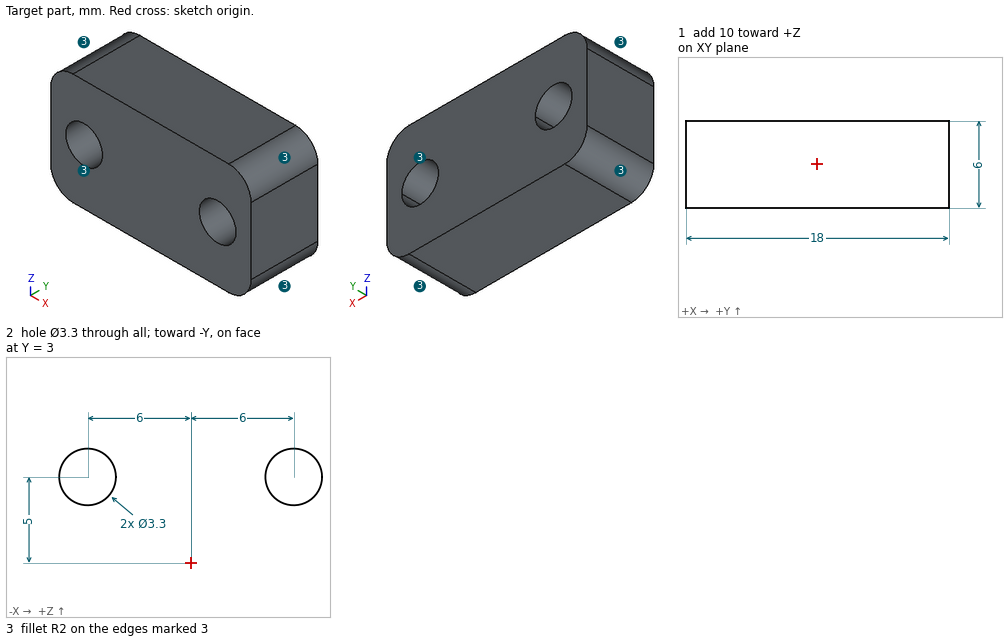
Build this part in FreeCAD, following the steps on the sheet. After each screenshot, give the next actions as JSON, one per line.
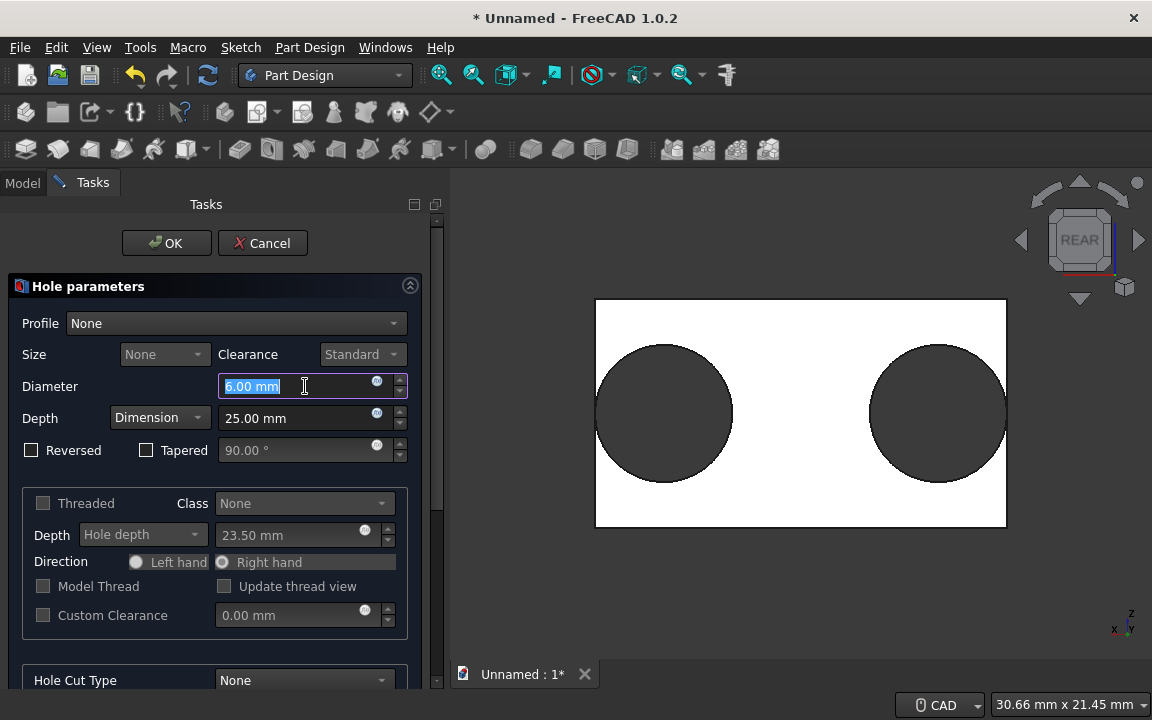
{"action": "type", "text": "3.3"}
{"action": "key", "text": "Tab"}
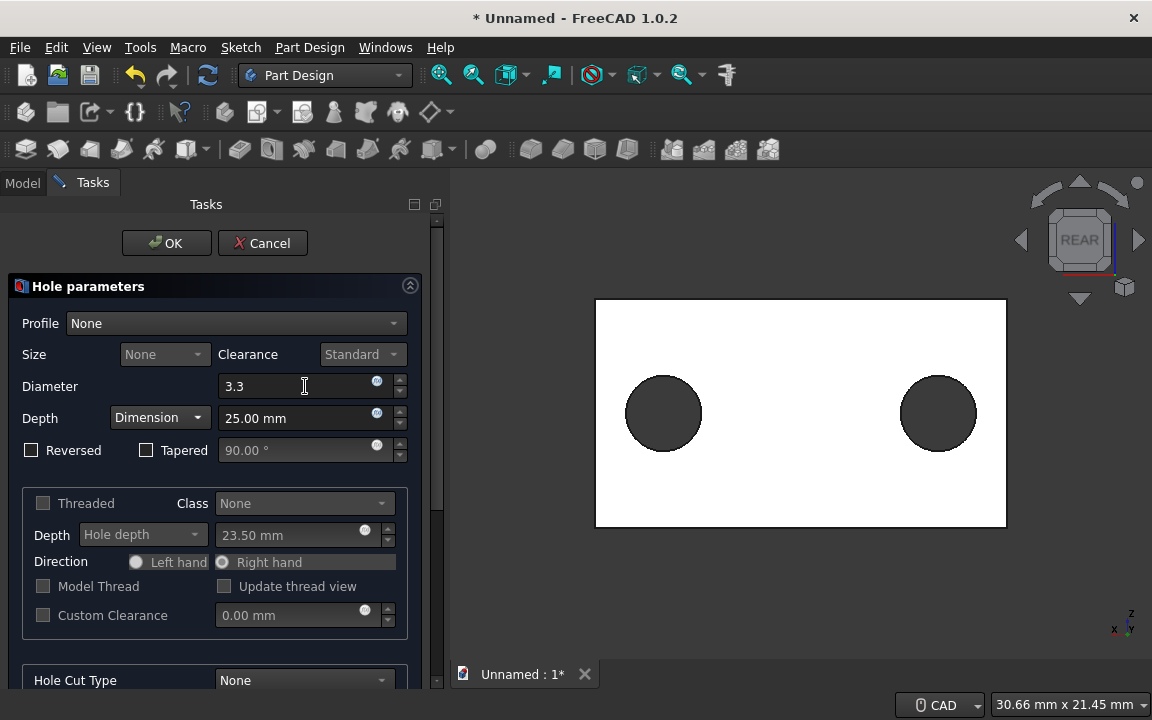
{"action": "left_click", "coordinate": [161, 418]}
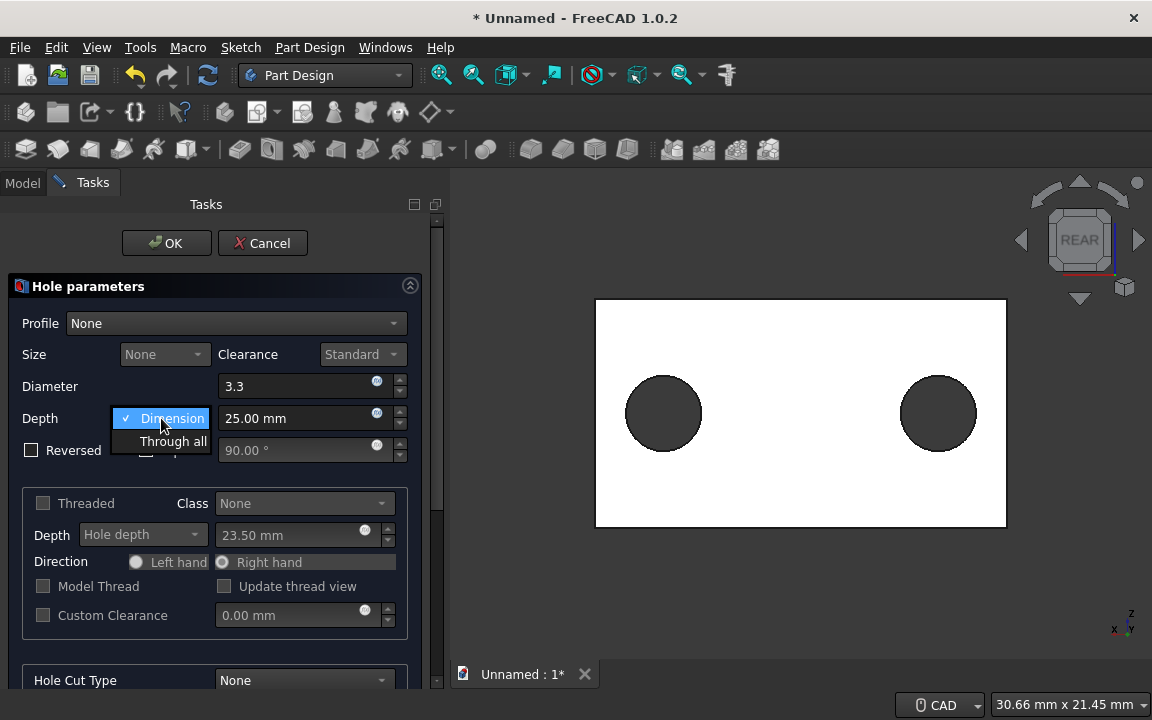
{"action": "left_click", "coordinate": [160, 442]}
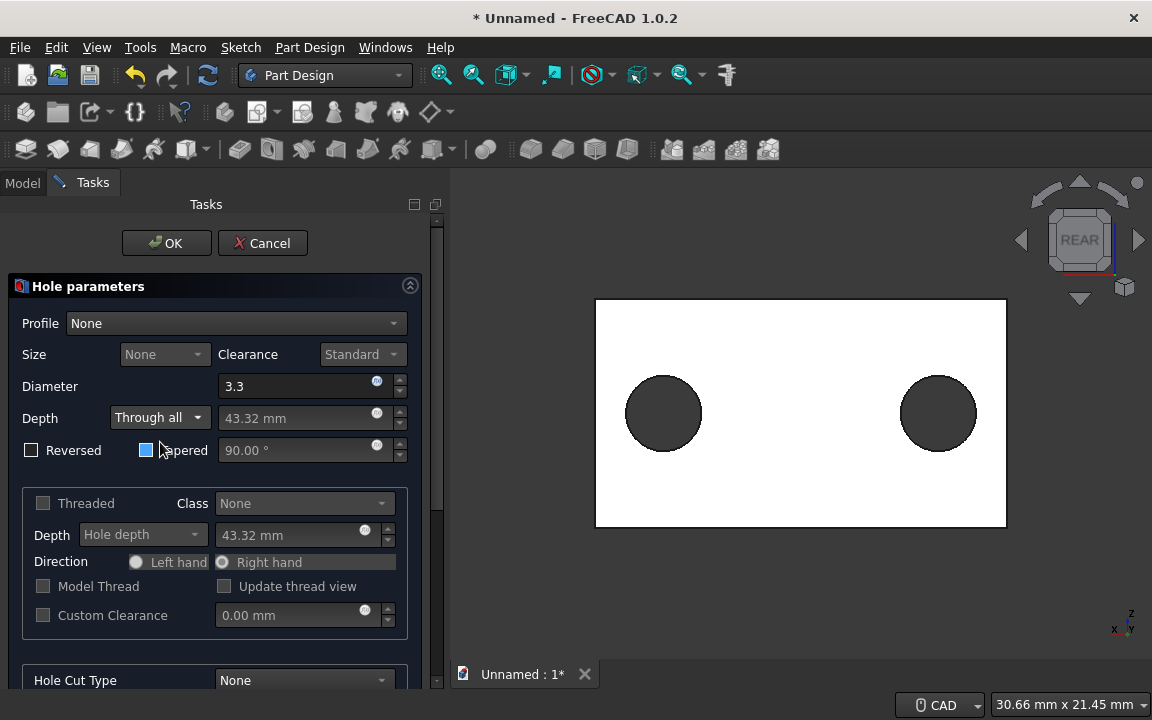
{"action": "left_click", "coordinate": [167, 243]}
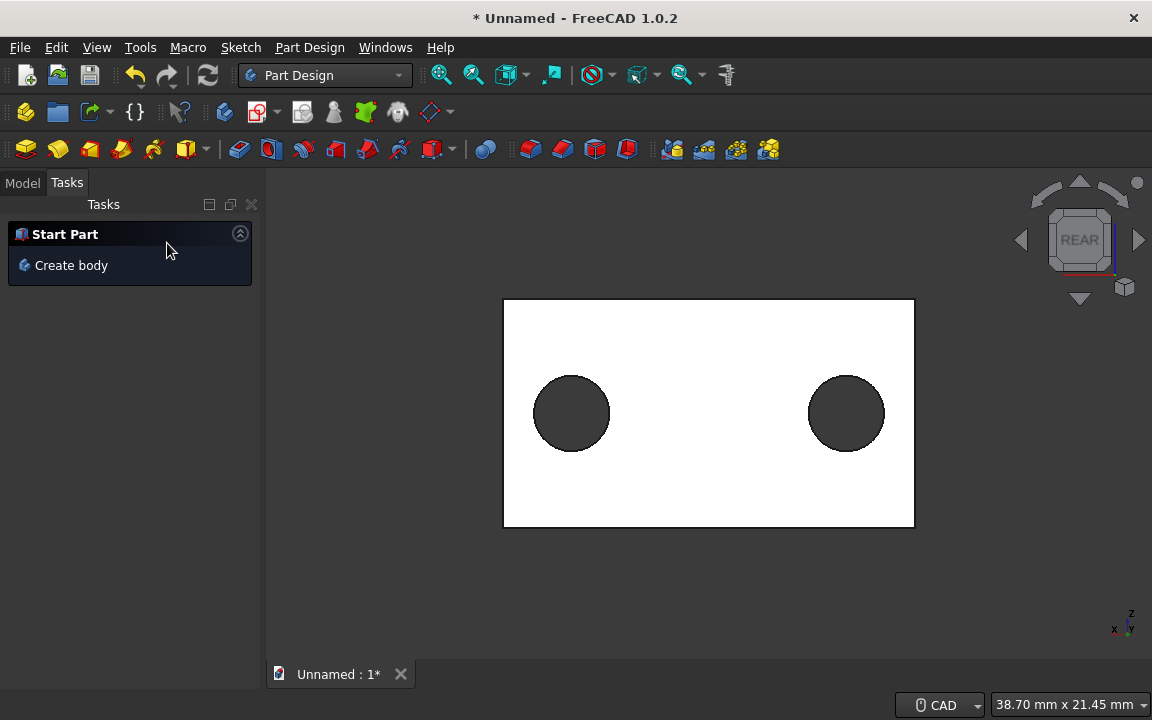
{"action": "key", "text": "0"}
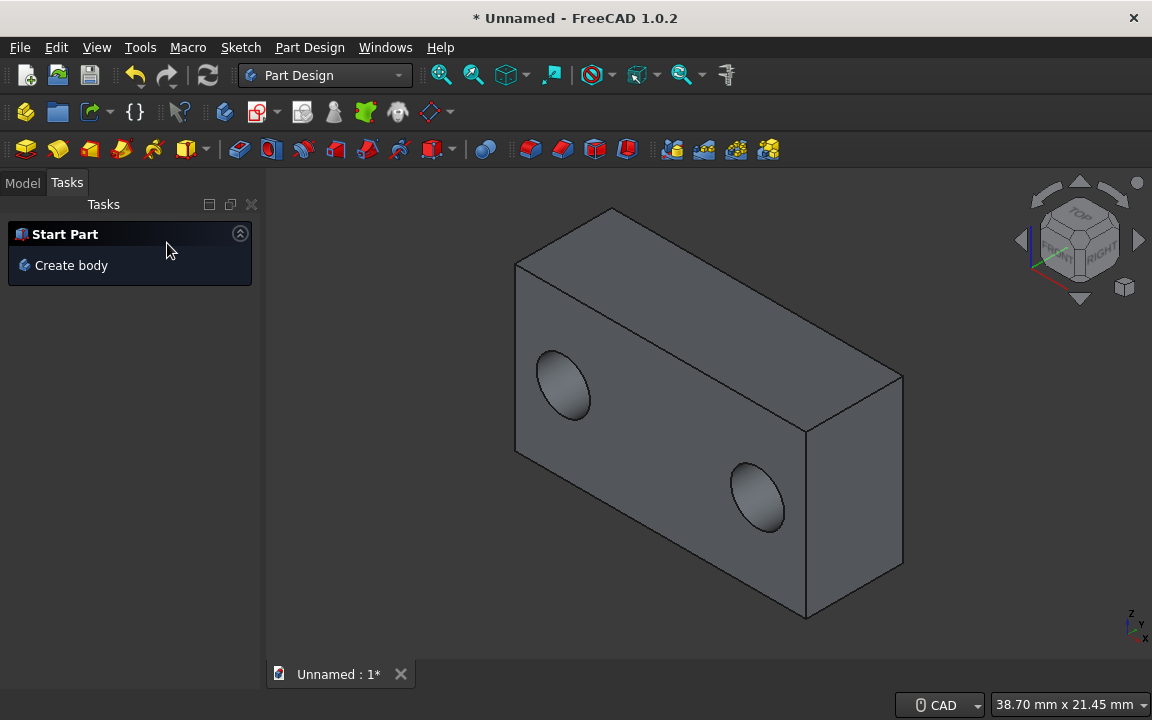
{"action": "left_click", "coordinate": [855, 403]}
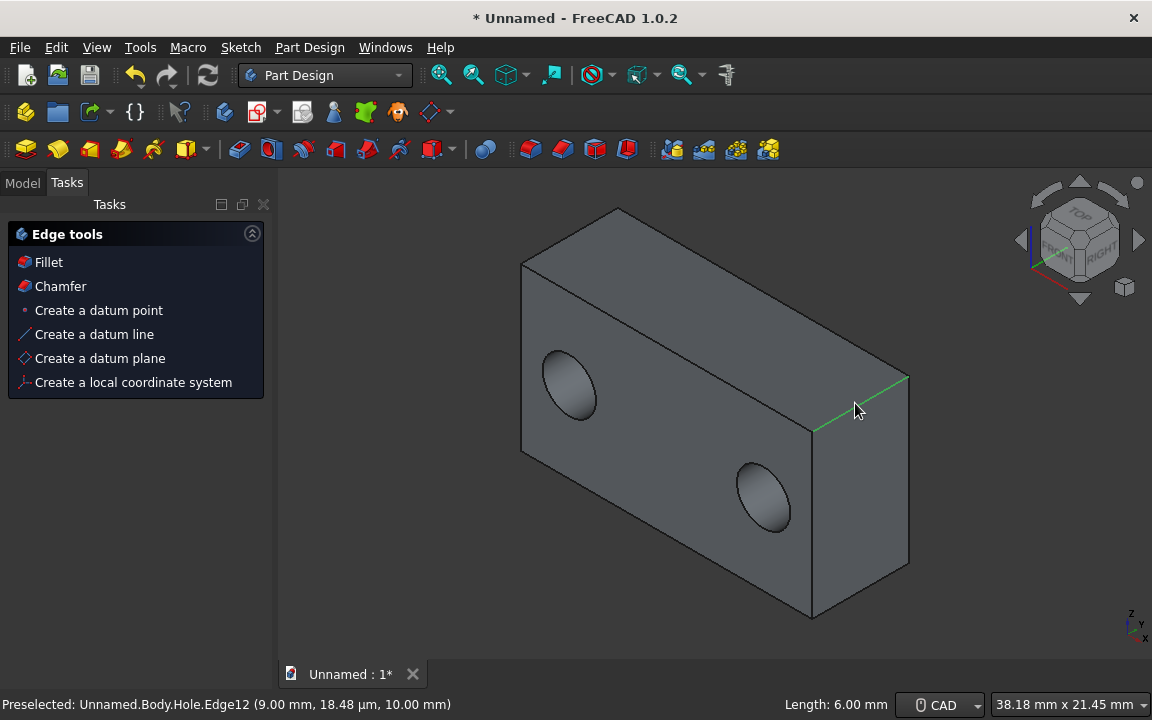
{"action": "key", "text": "2"}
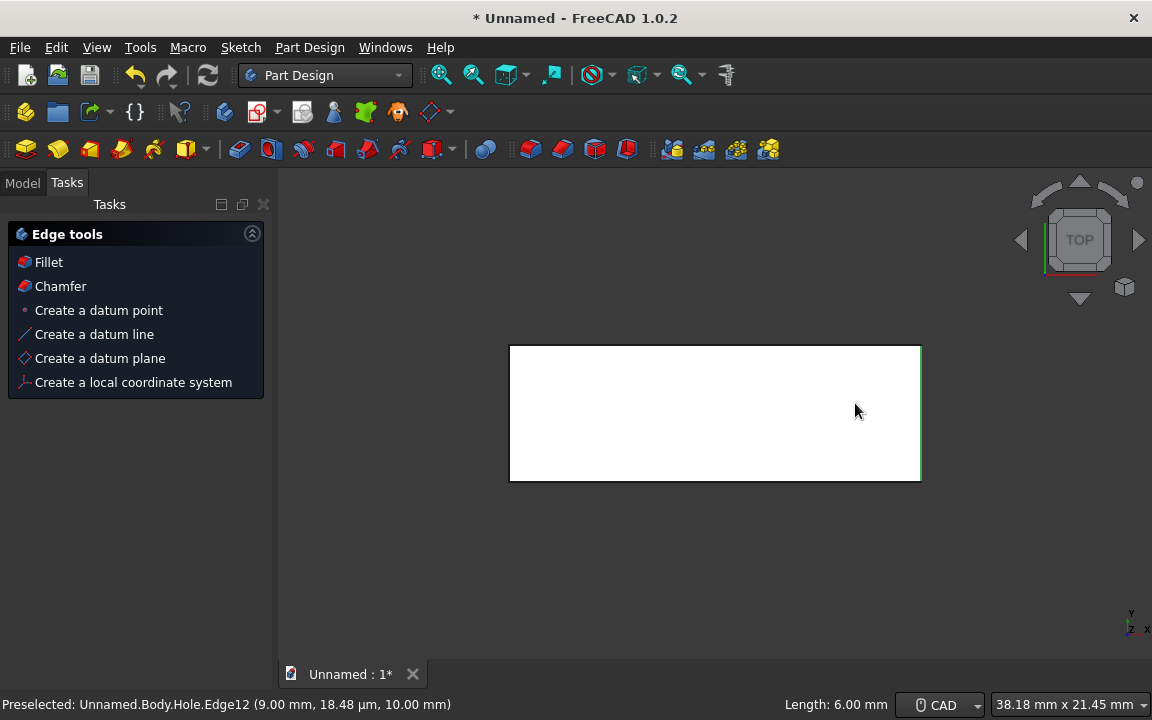
{"action": "left_click", "coordinate": [509, 412], "text": "ctrl"}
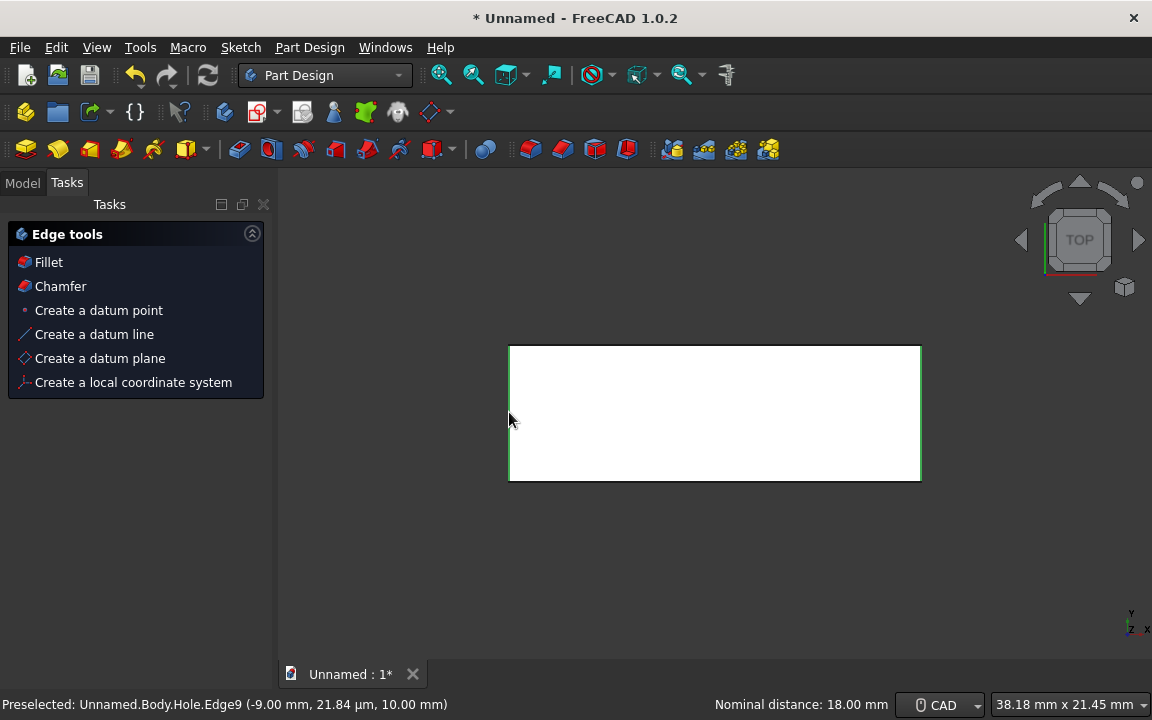
{"action": "key", "text": "1"}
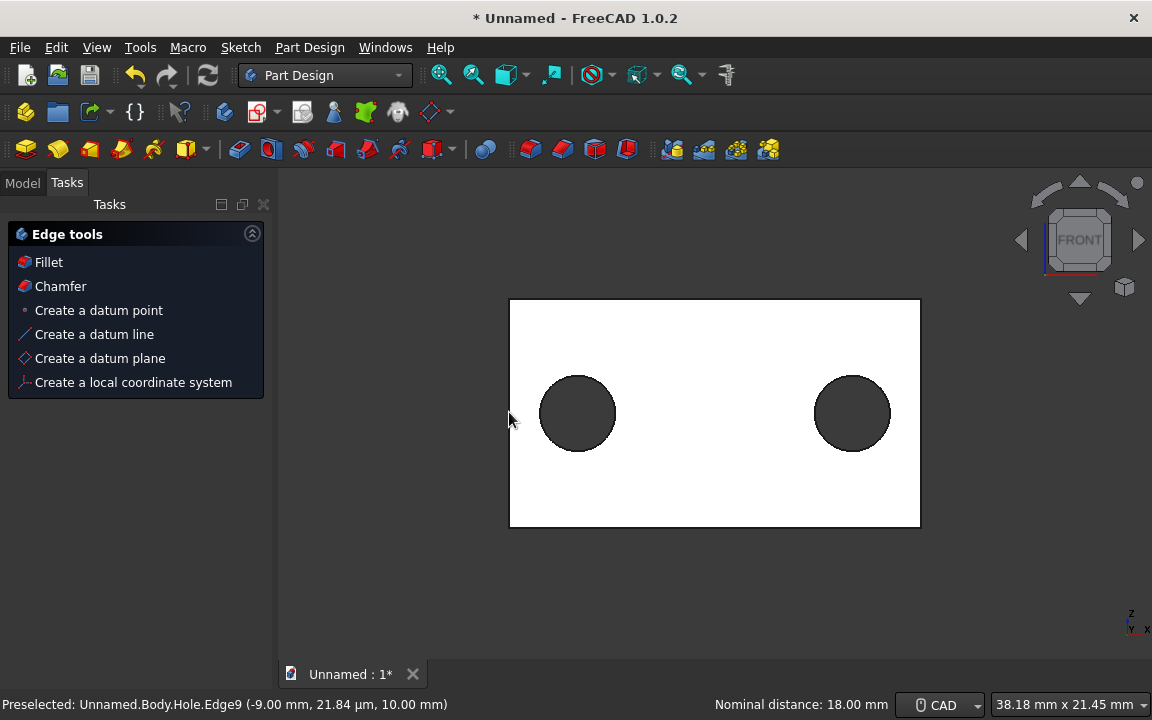
{"action": "key", "text": "3"}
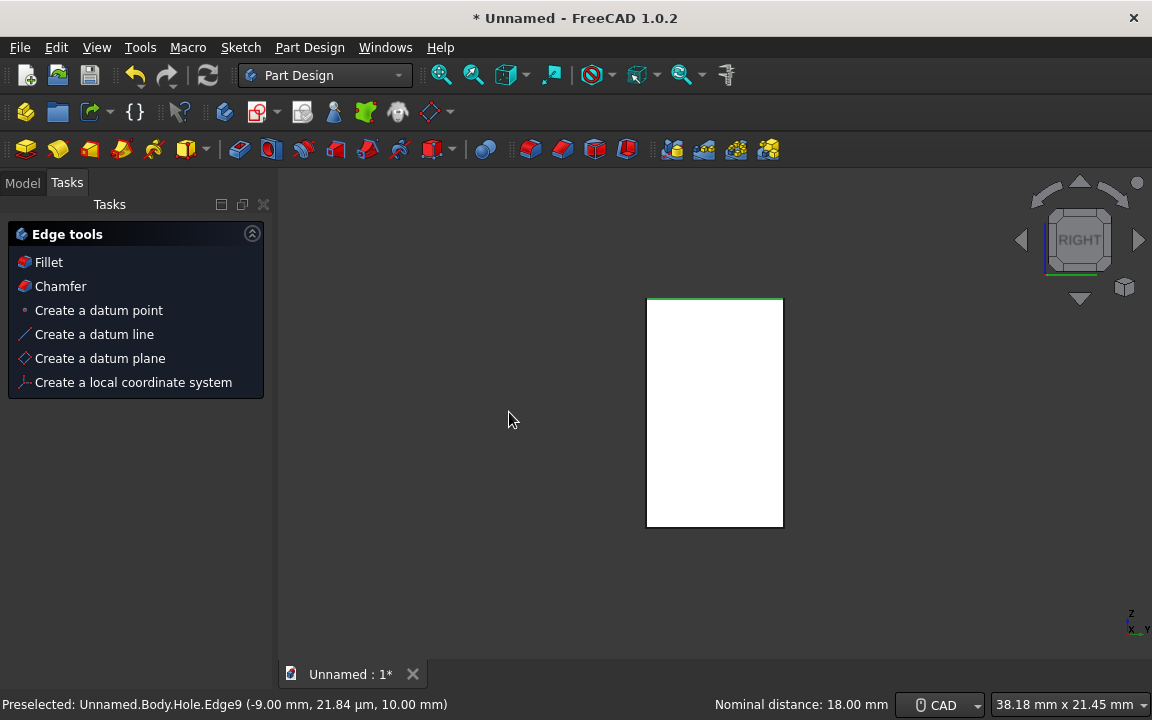
{"action": "left_click", "coordinate": [715, 527], "text": "ctrl"}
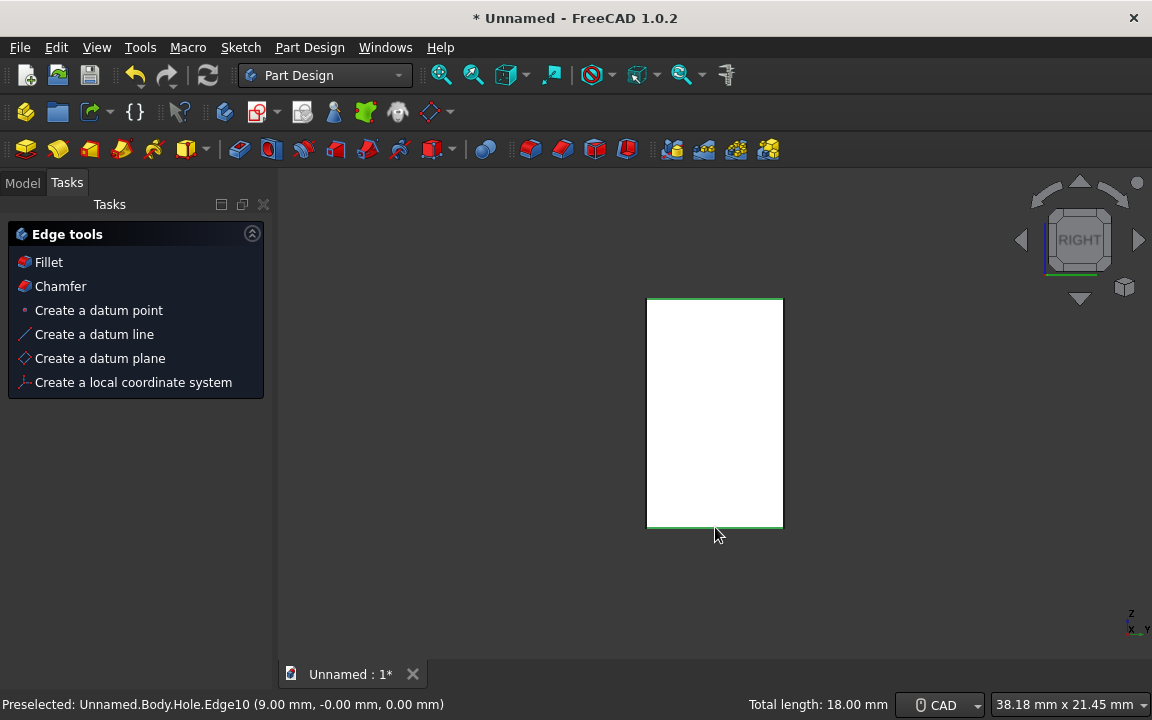
{"action": "key", "text": "5"}